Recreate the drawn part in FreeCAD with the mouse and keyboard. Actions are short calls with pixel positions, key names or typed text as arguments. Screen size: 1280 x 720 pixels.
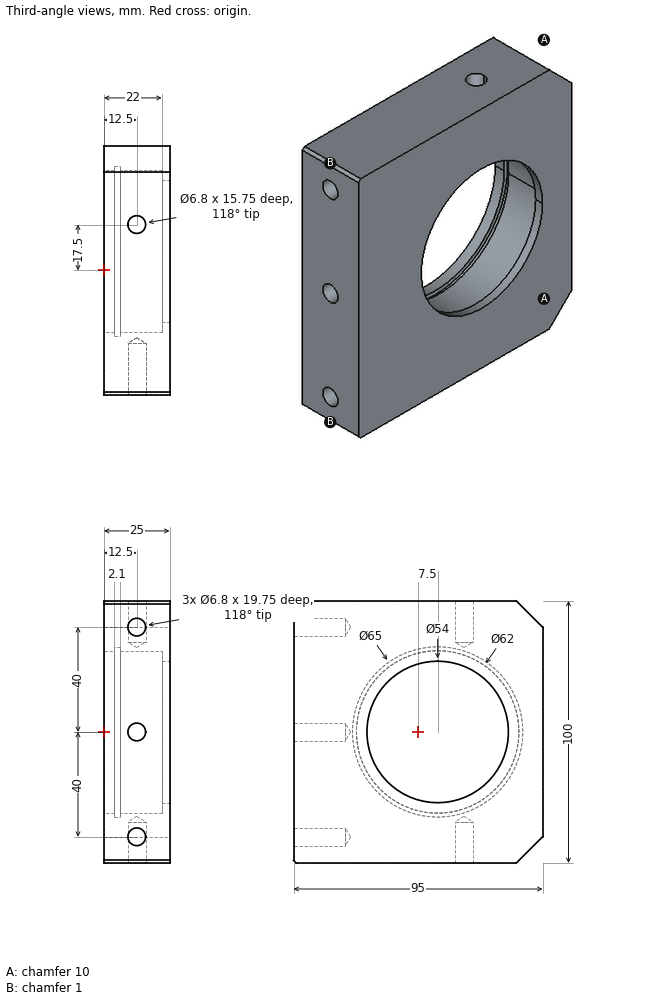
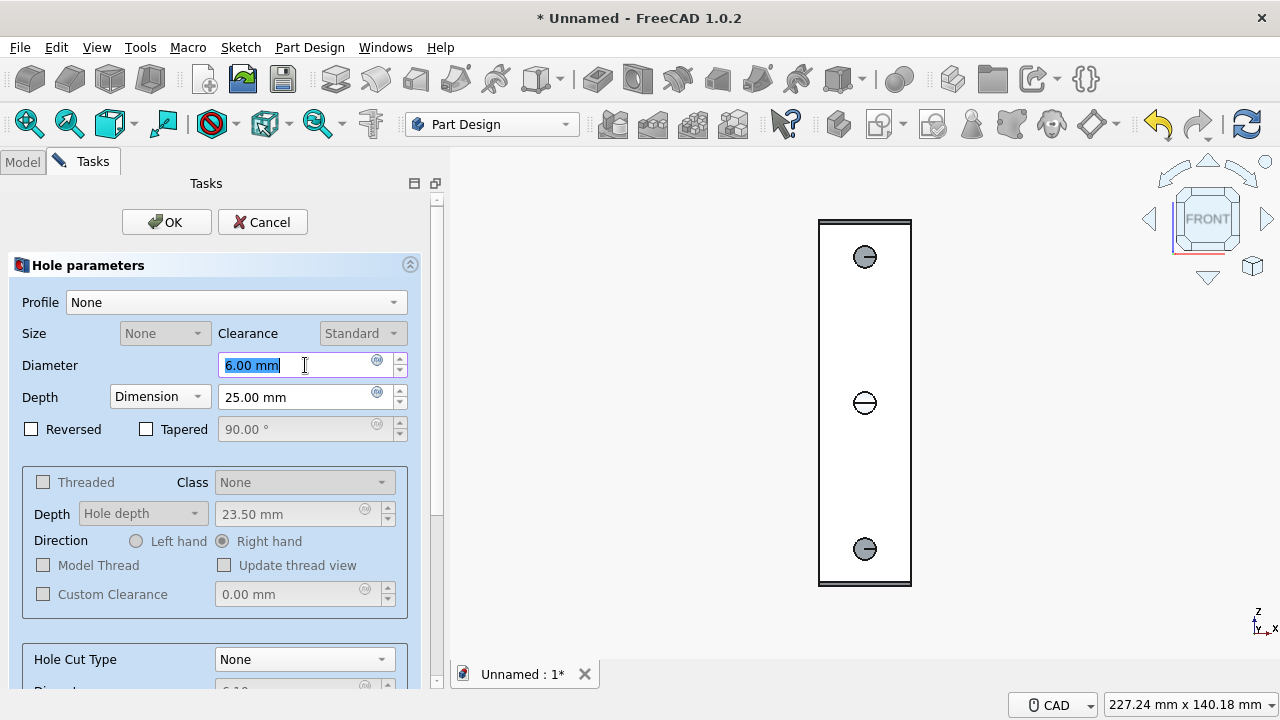
text(6.8)
key(Tab)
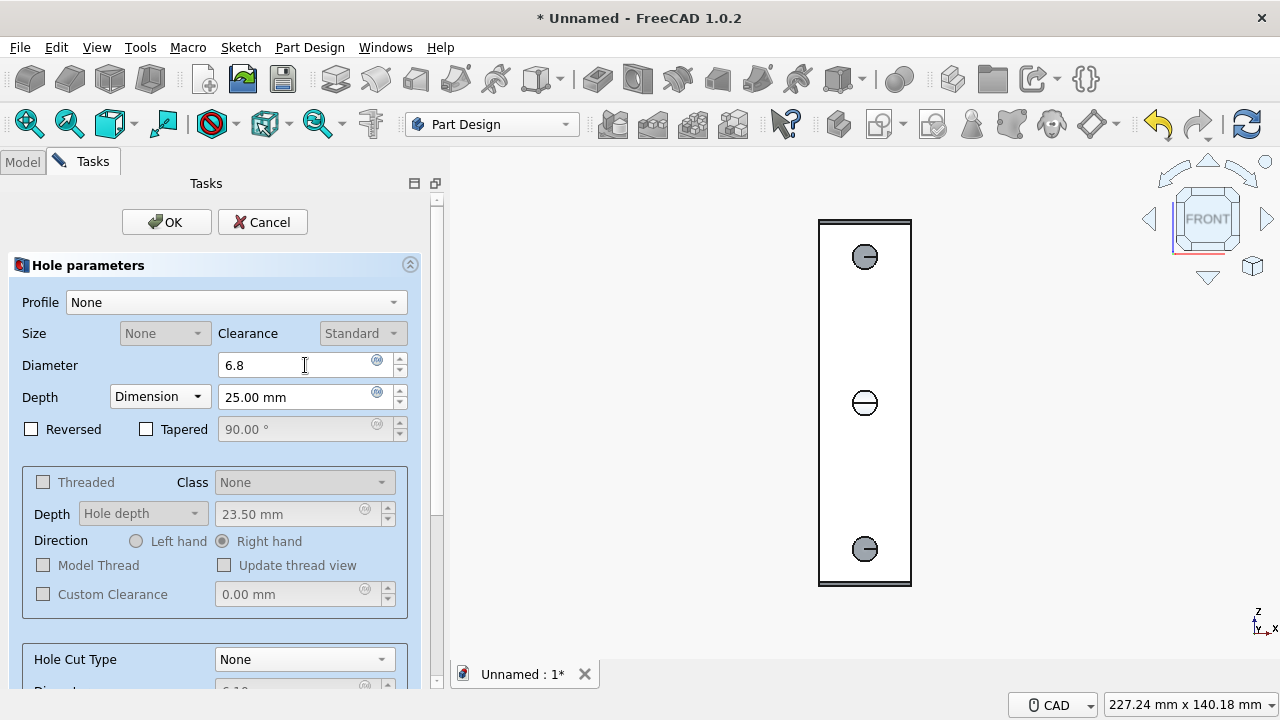
triple_click(305, 397)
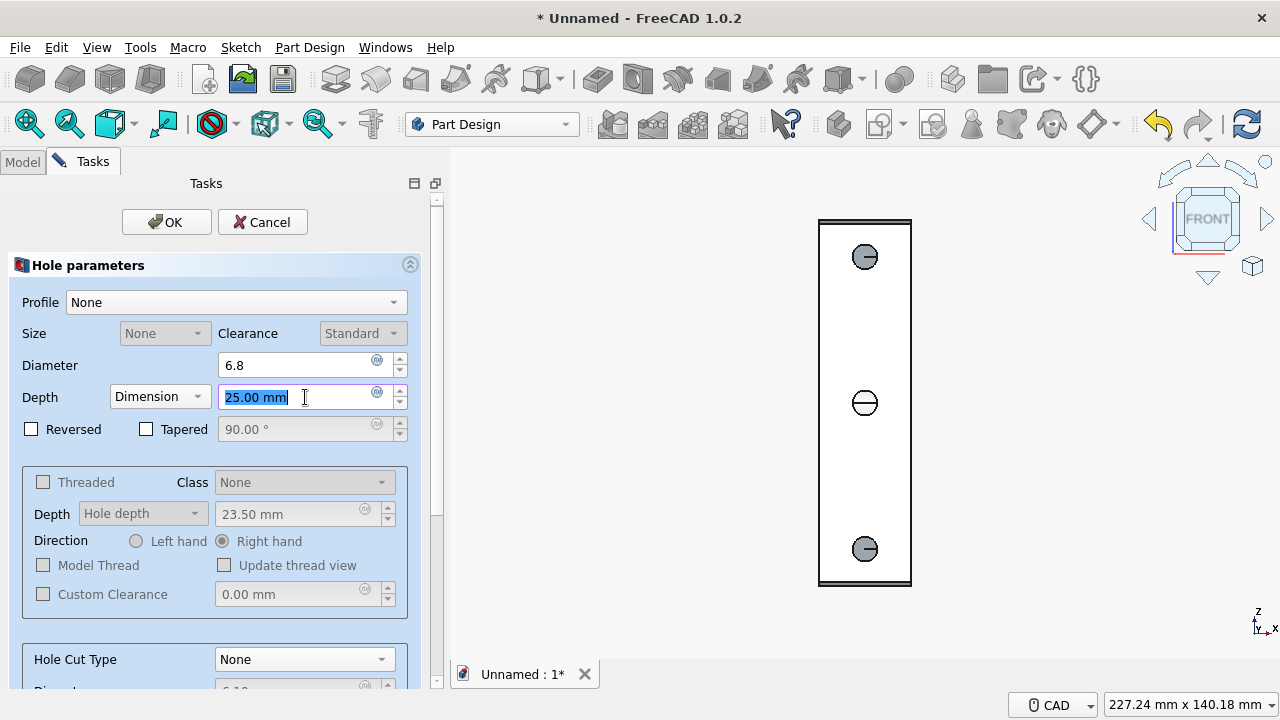
text(19.75)
key(Tab)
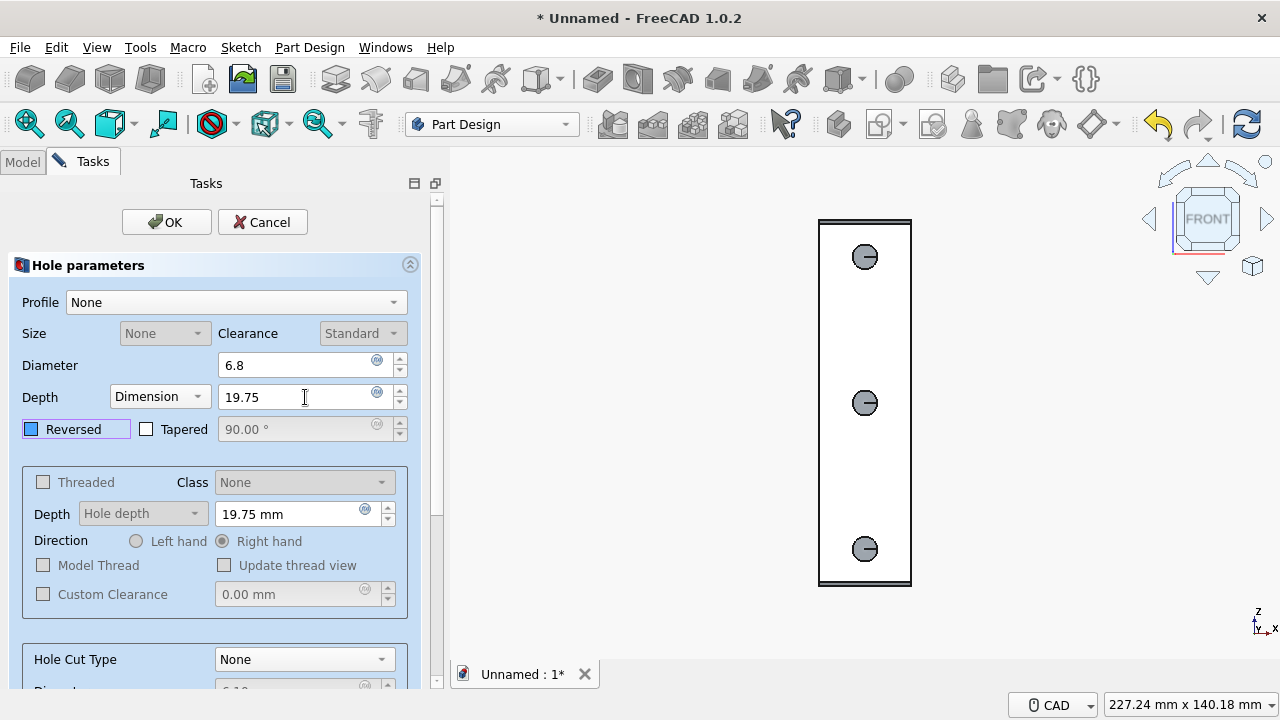
click(167, 222)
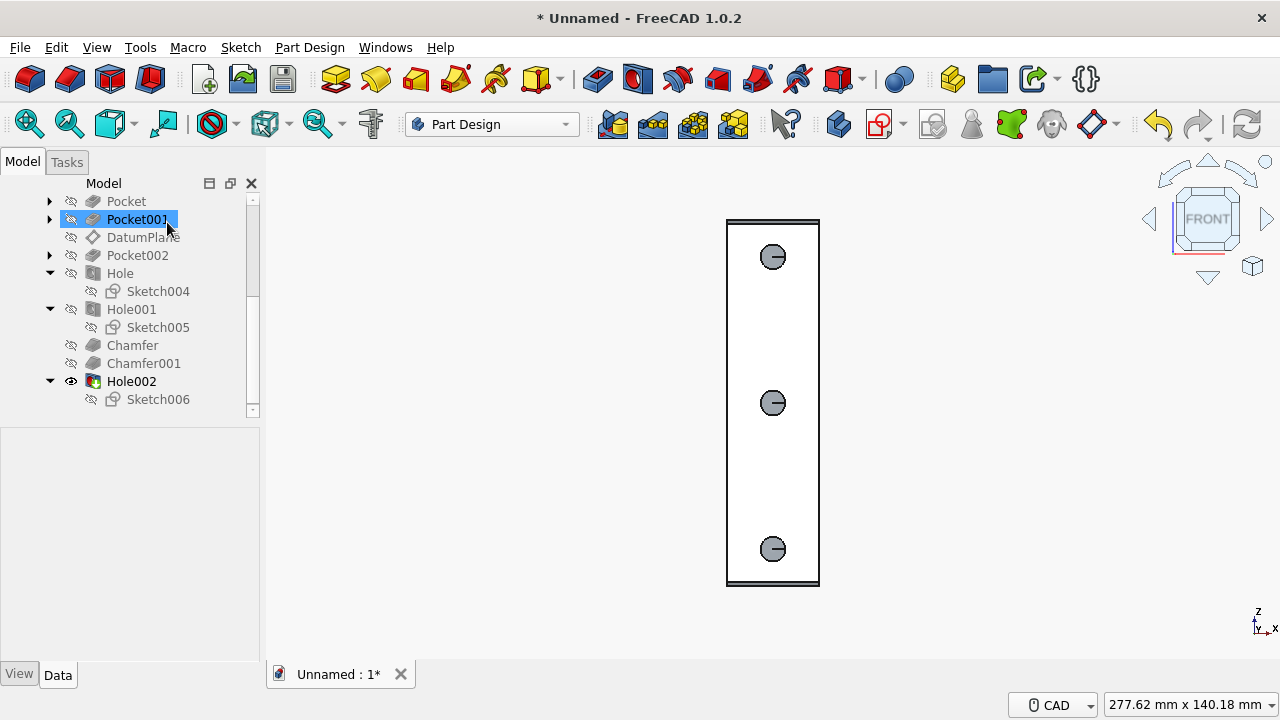
key(0)